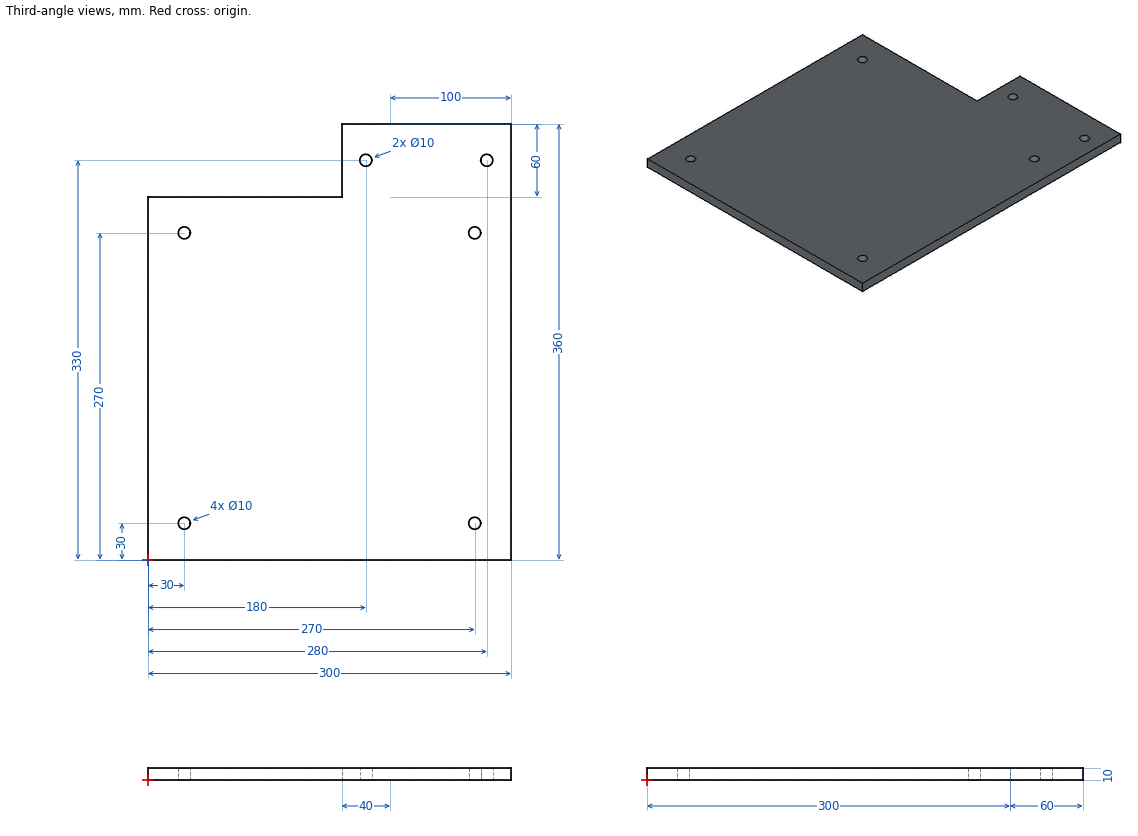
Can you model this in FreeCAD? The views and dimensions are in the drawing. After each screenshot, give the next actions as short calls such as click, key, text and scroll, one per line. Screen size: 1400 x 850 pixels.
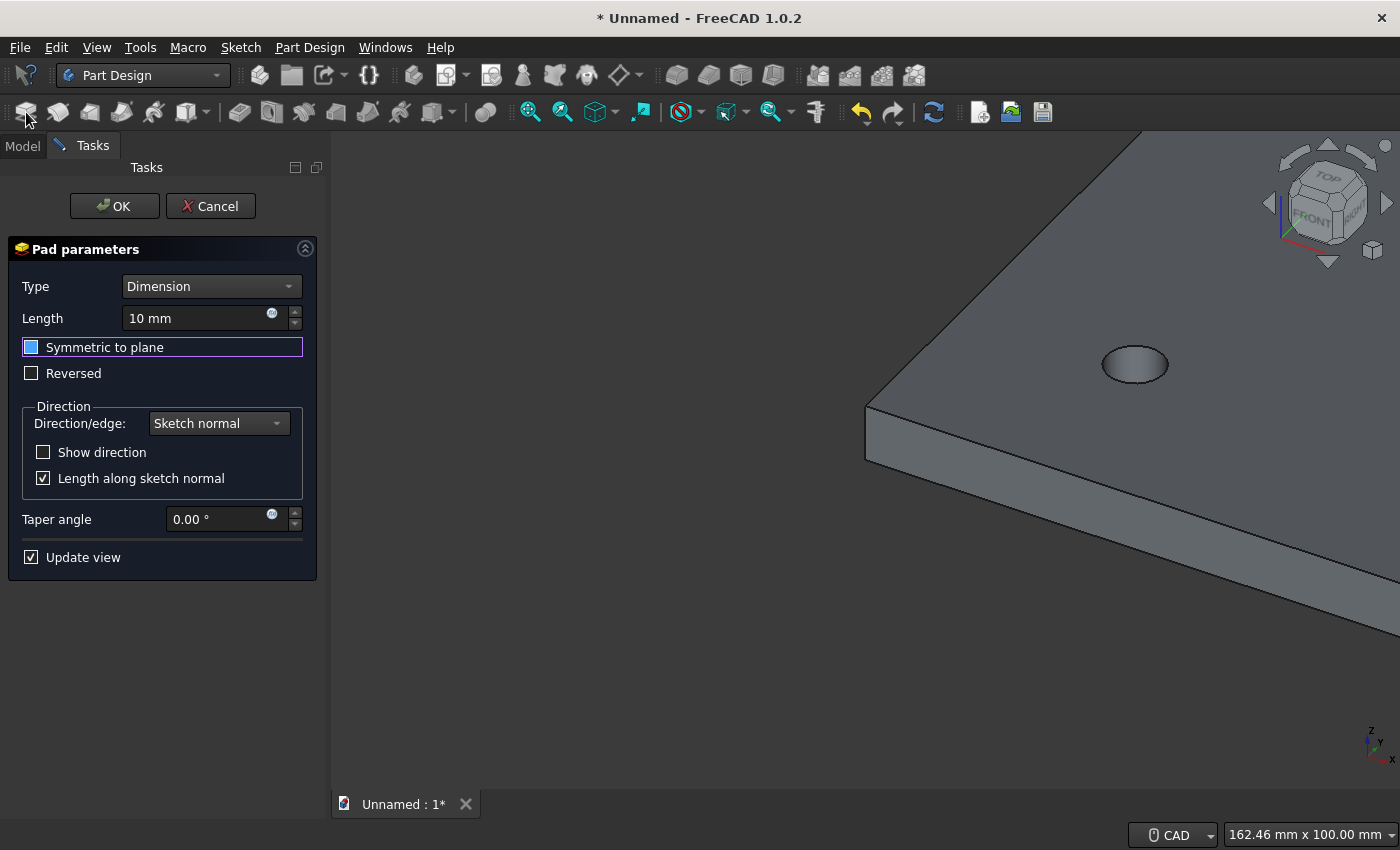
click(115, 206)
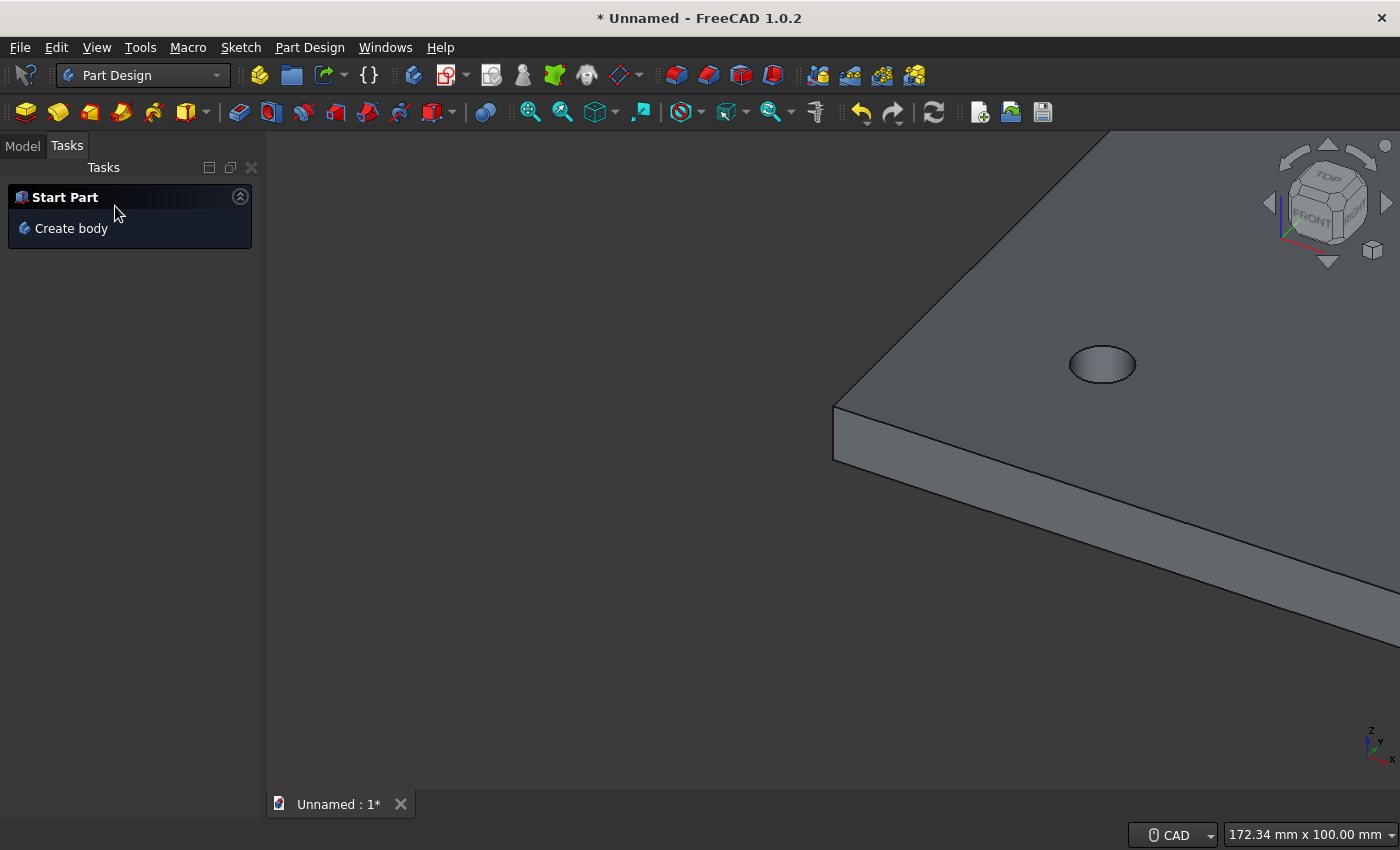
click(532, 112)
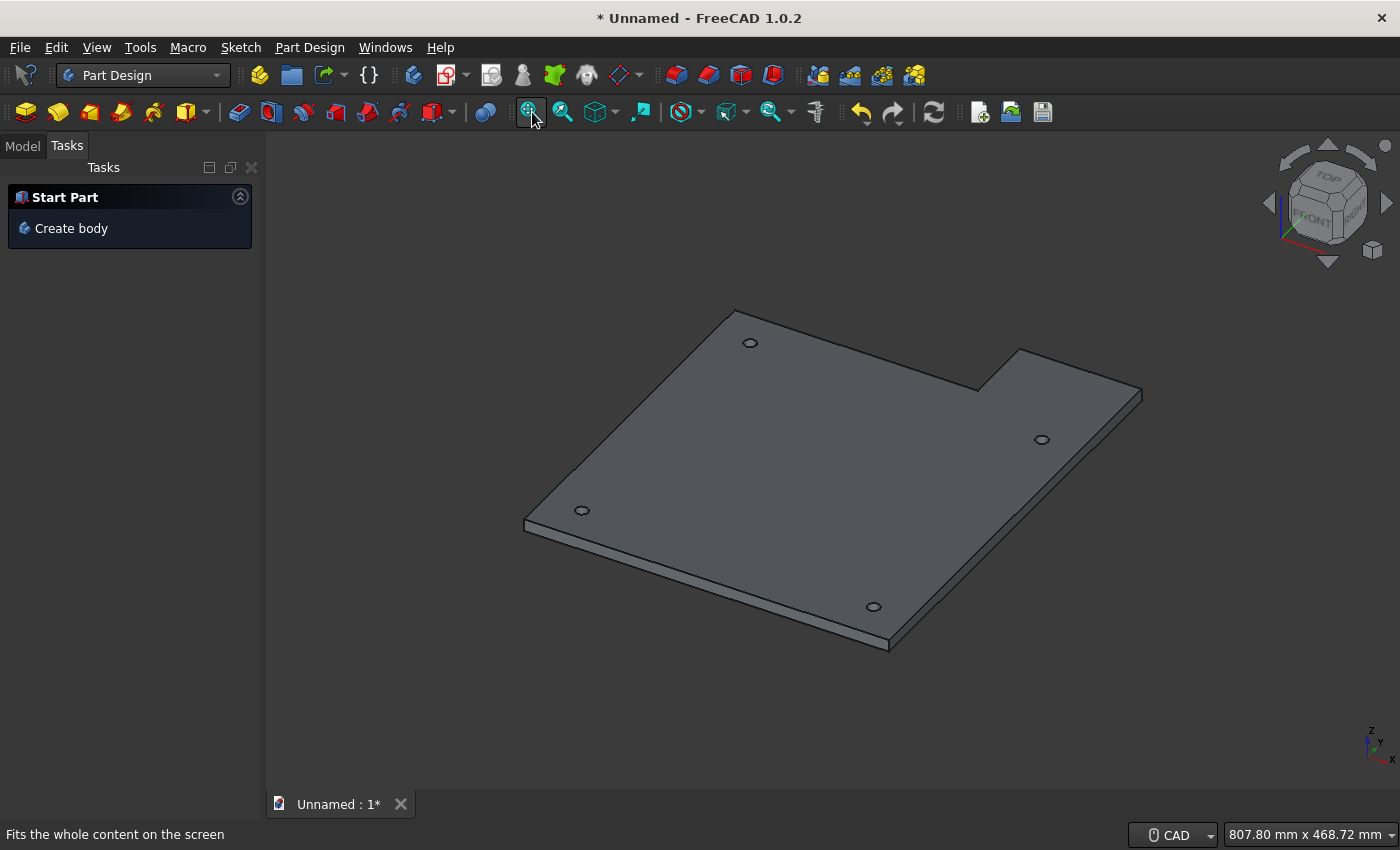
key(6)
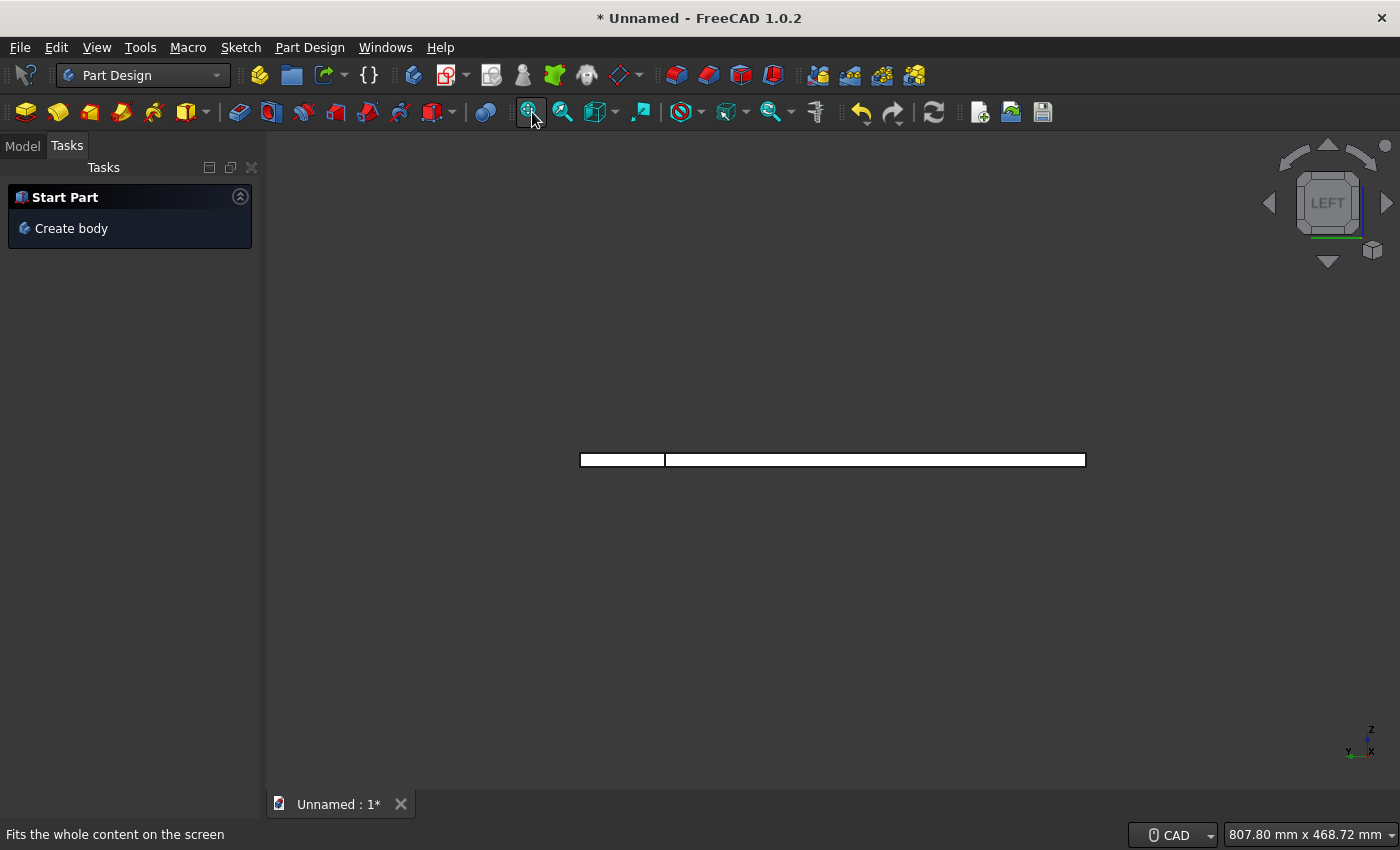
click(532, 112)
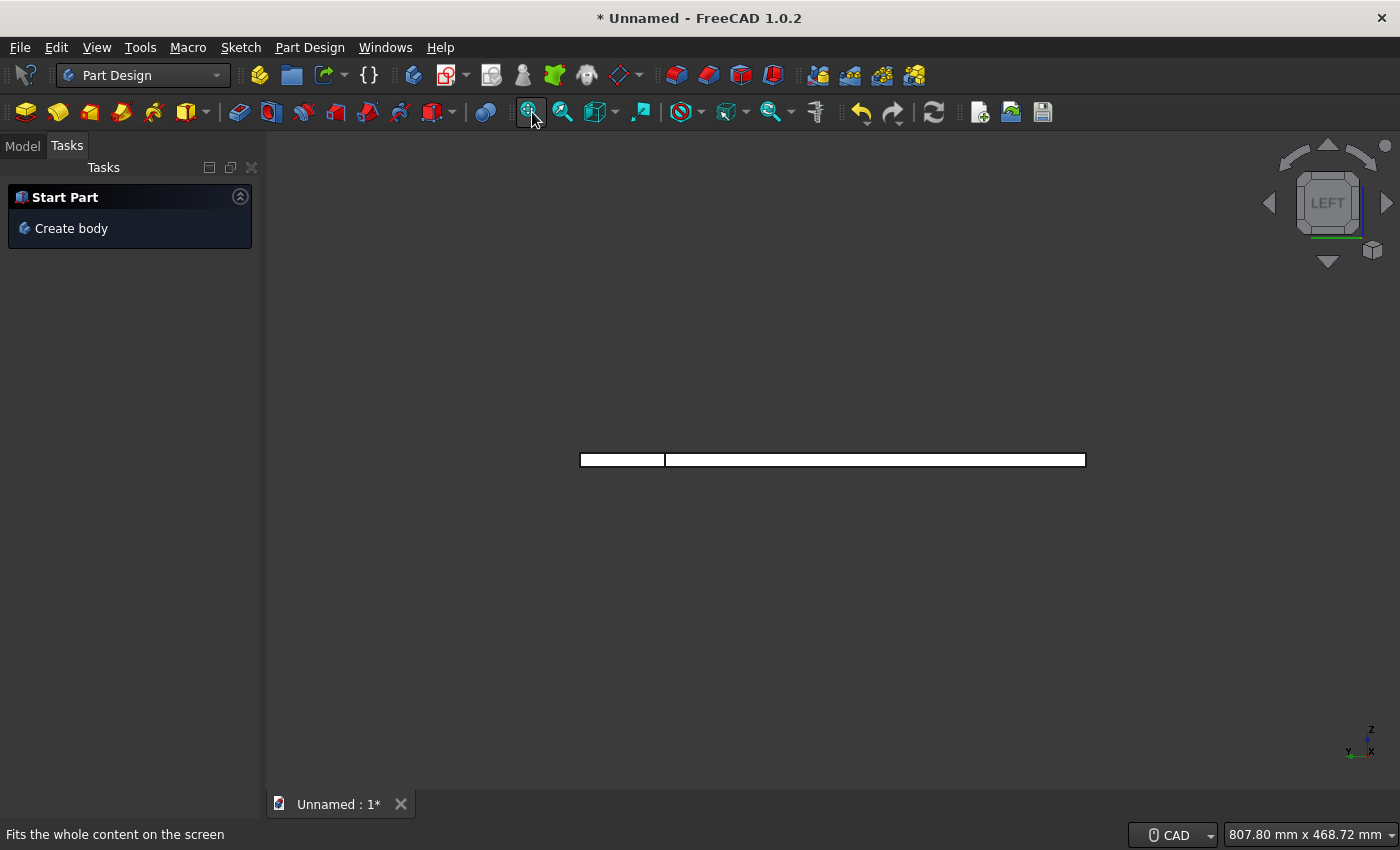
key(2)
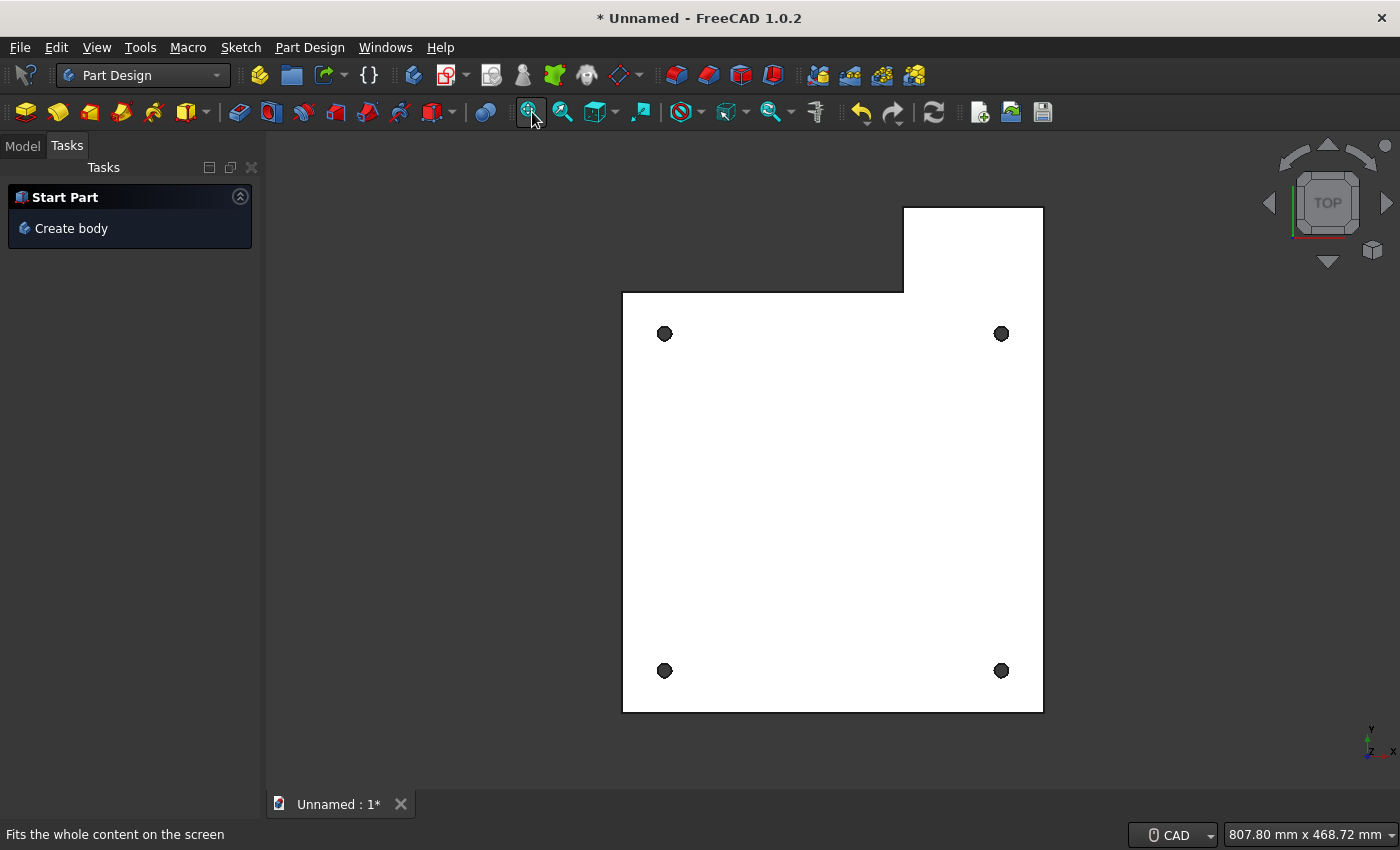
key(1)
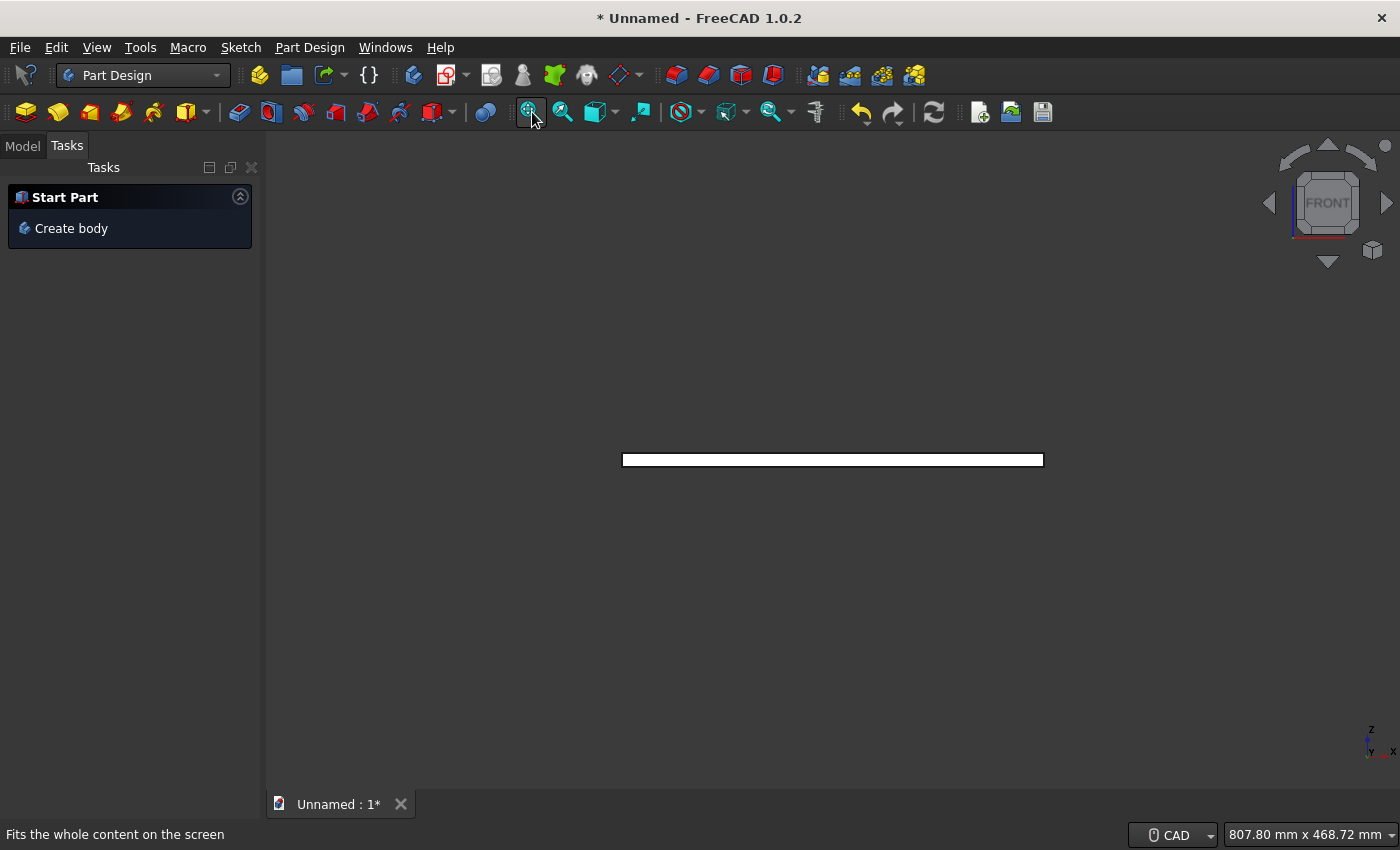
click(532, 112)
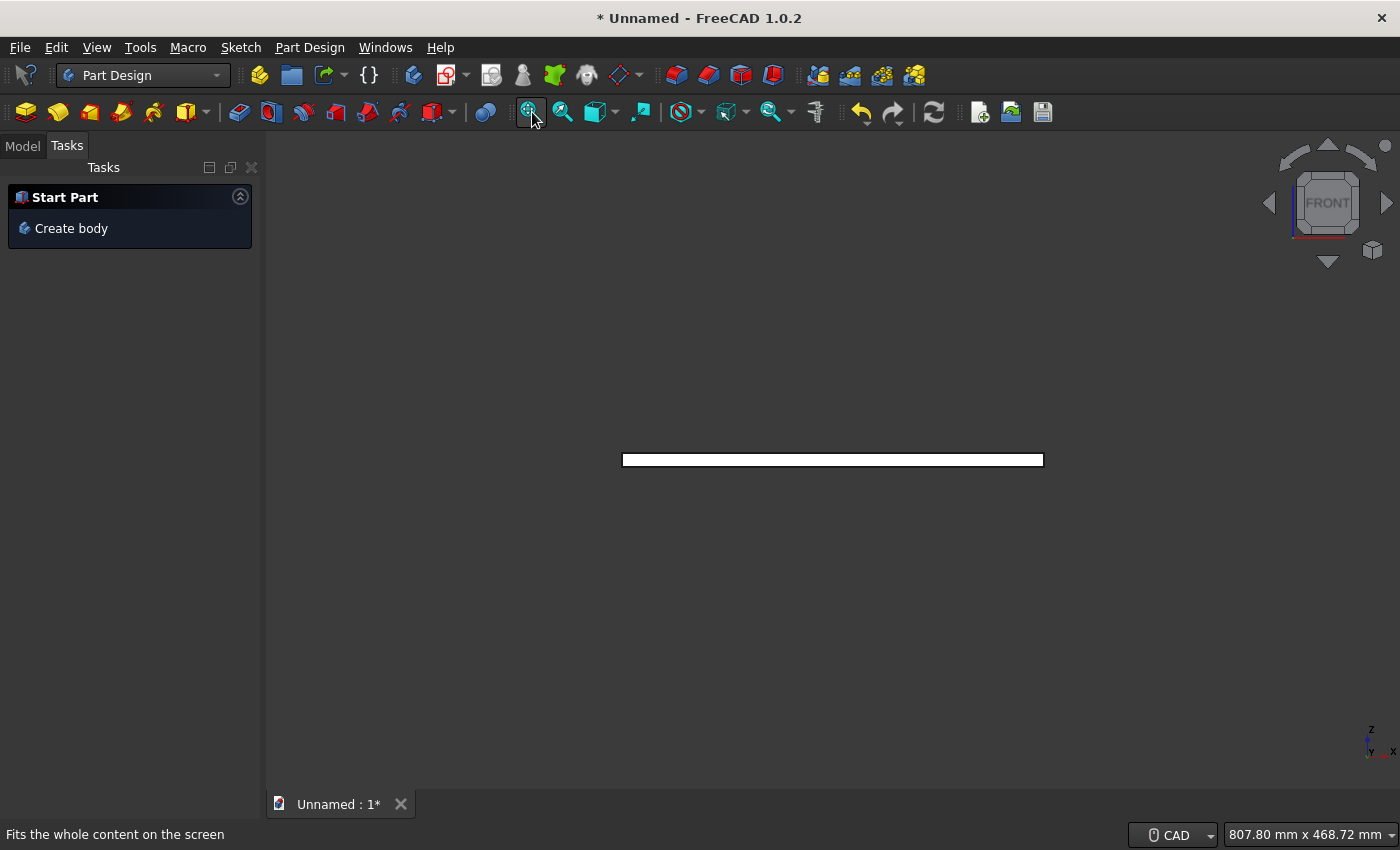
click(23, 145)